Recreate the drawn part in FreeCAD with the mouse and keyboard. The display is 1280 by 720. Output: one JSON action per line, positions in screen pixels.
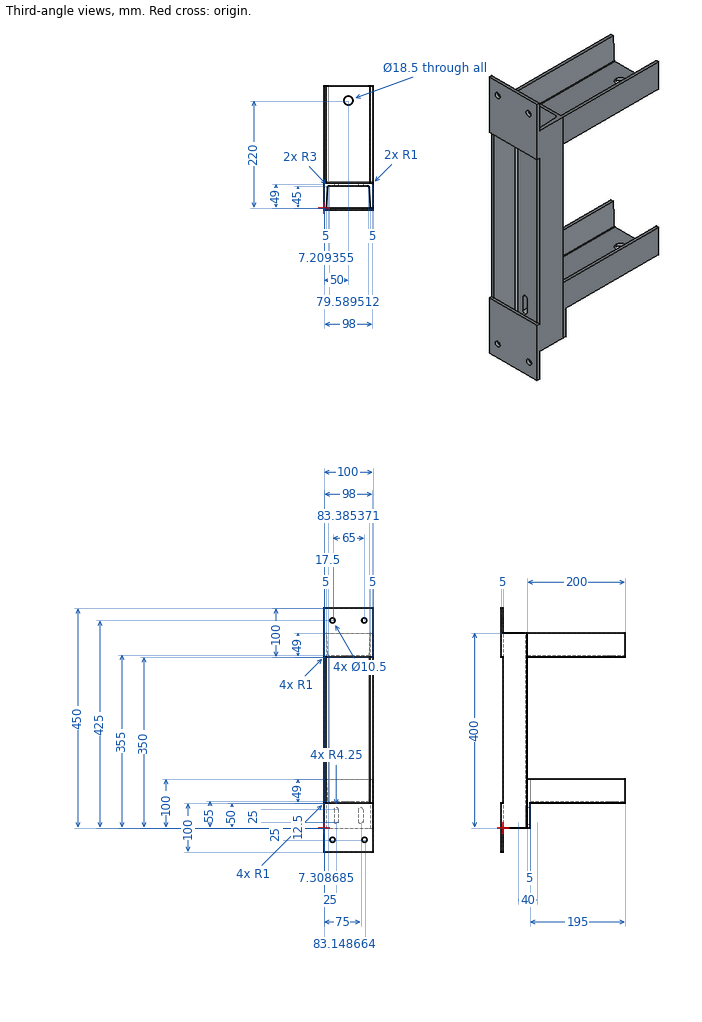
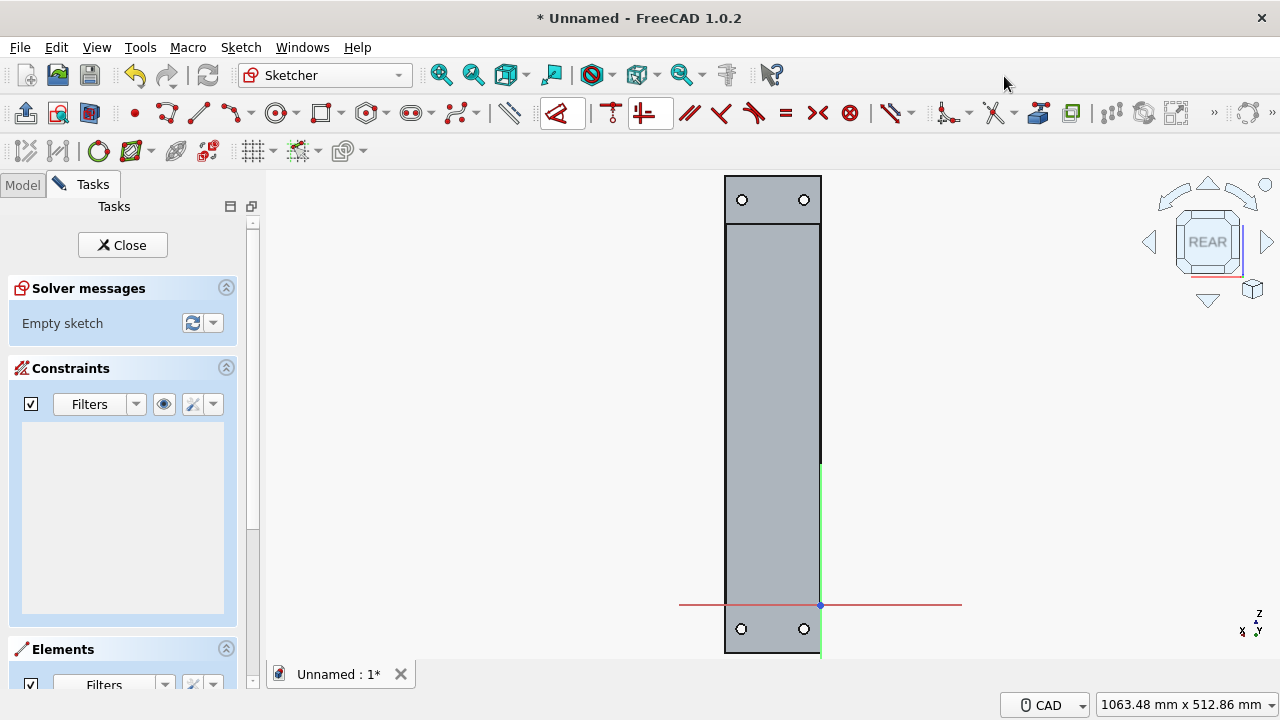
{"action": "scroll", "coordinate": [787, 215], "scroll_direction": "up", "scroll_amount": 9}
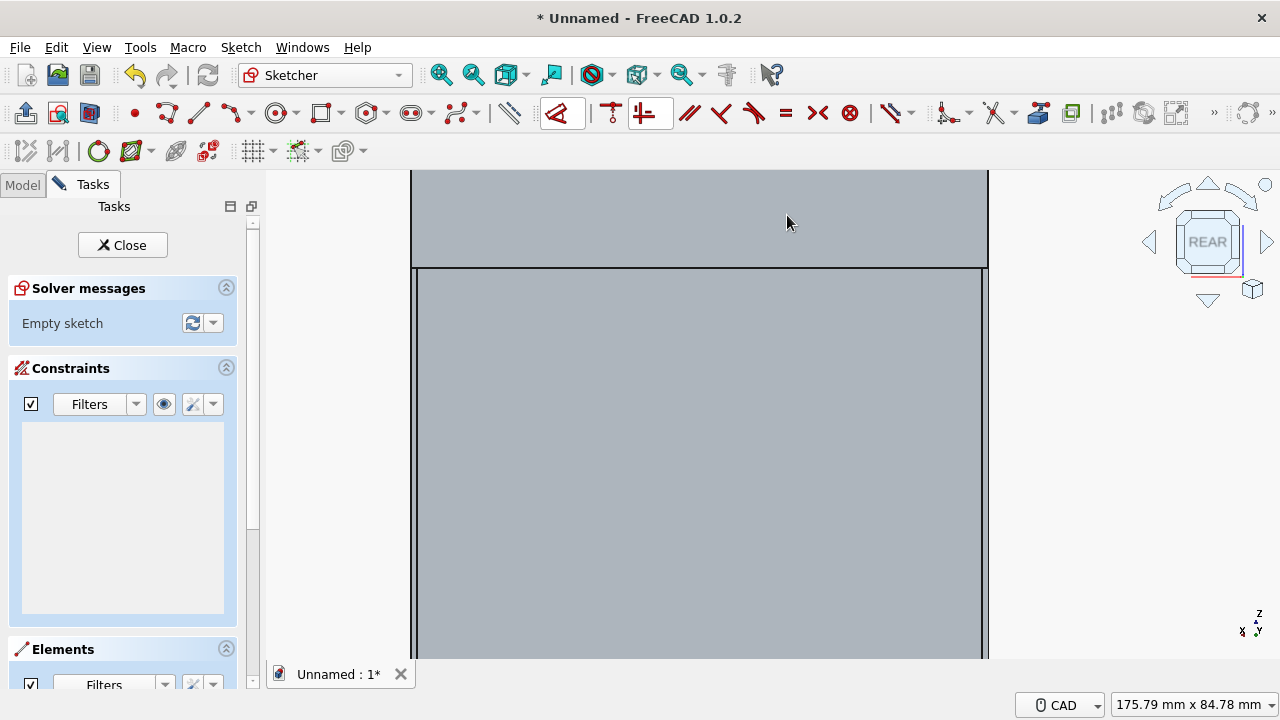
{"action": "key", "text": "g l"}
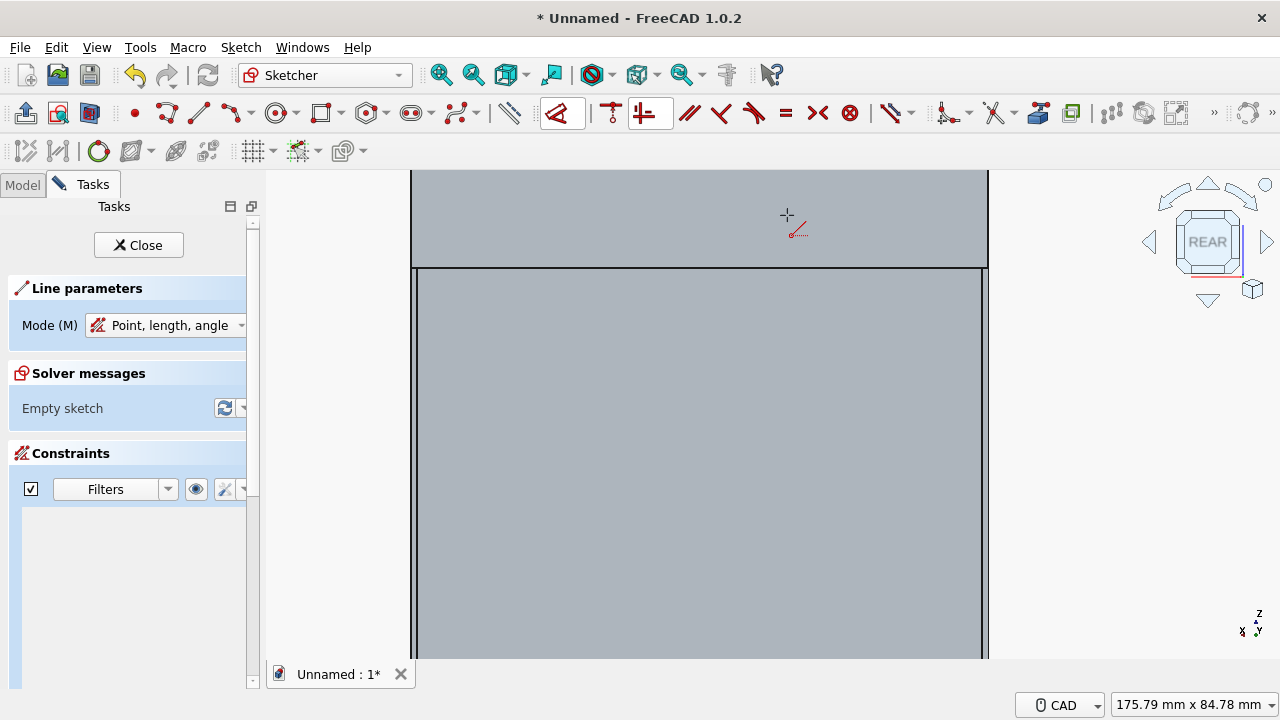
{"action": "left_click", "coordinate": [417, 556]}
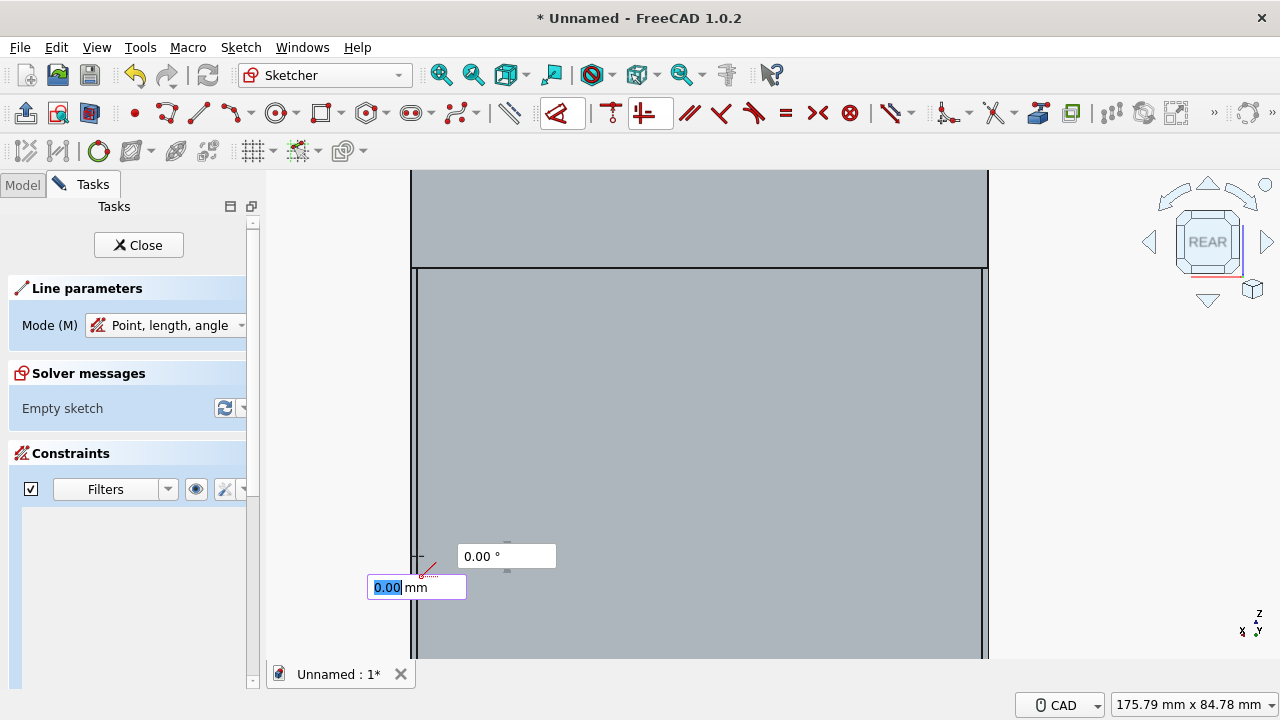
{"action": "scroll", "coordinate": [982, 556], "scroll_direction": "up", "scroll_amount": 6}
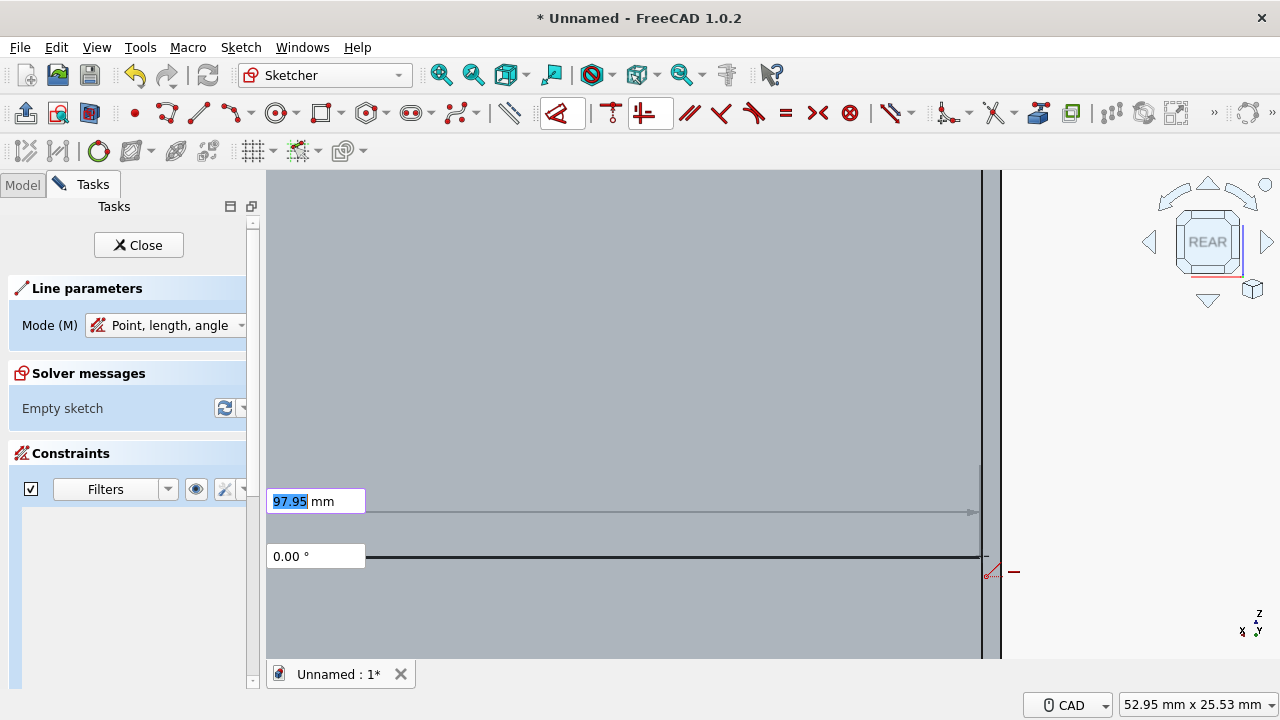
{"action": "left_click", "coordinate": [982, 554]}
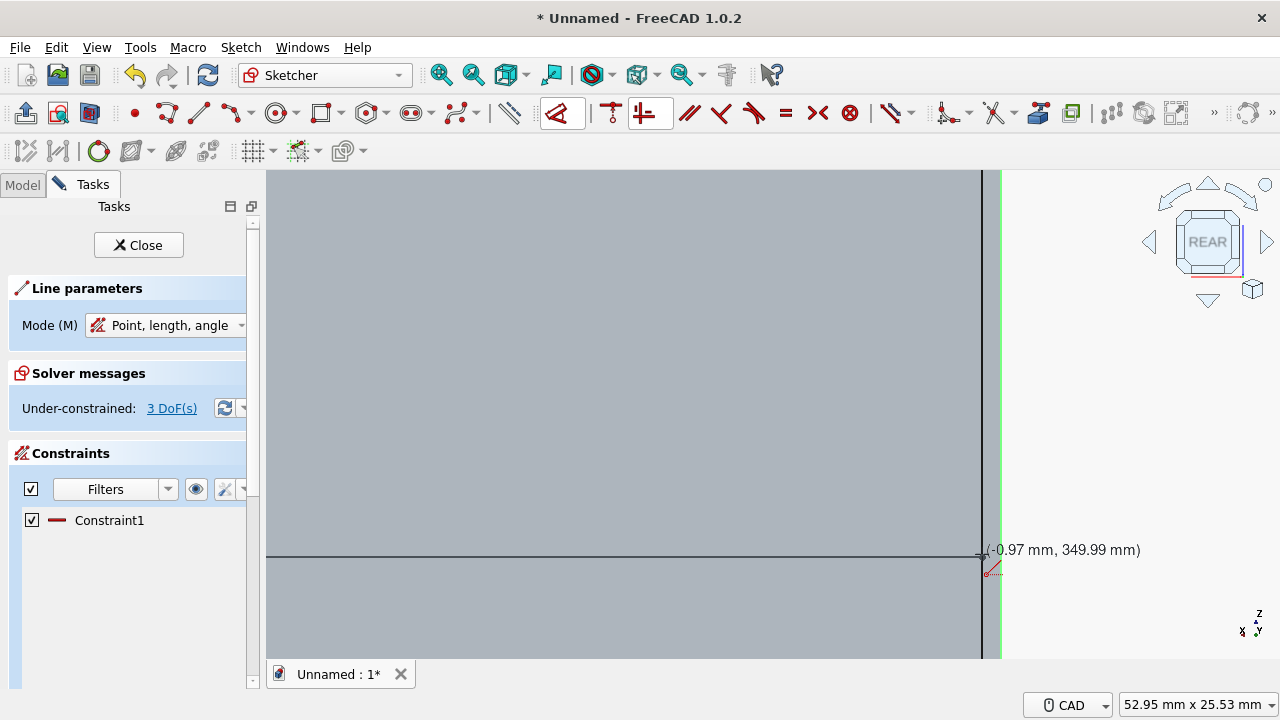
{"action": "key", "text": "g m"}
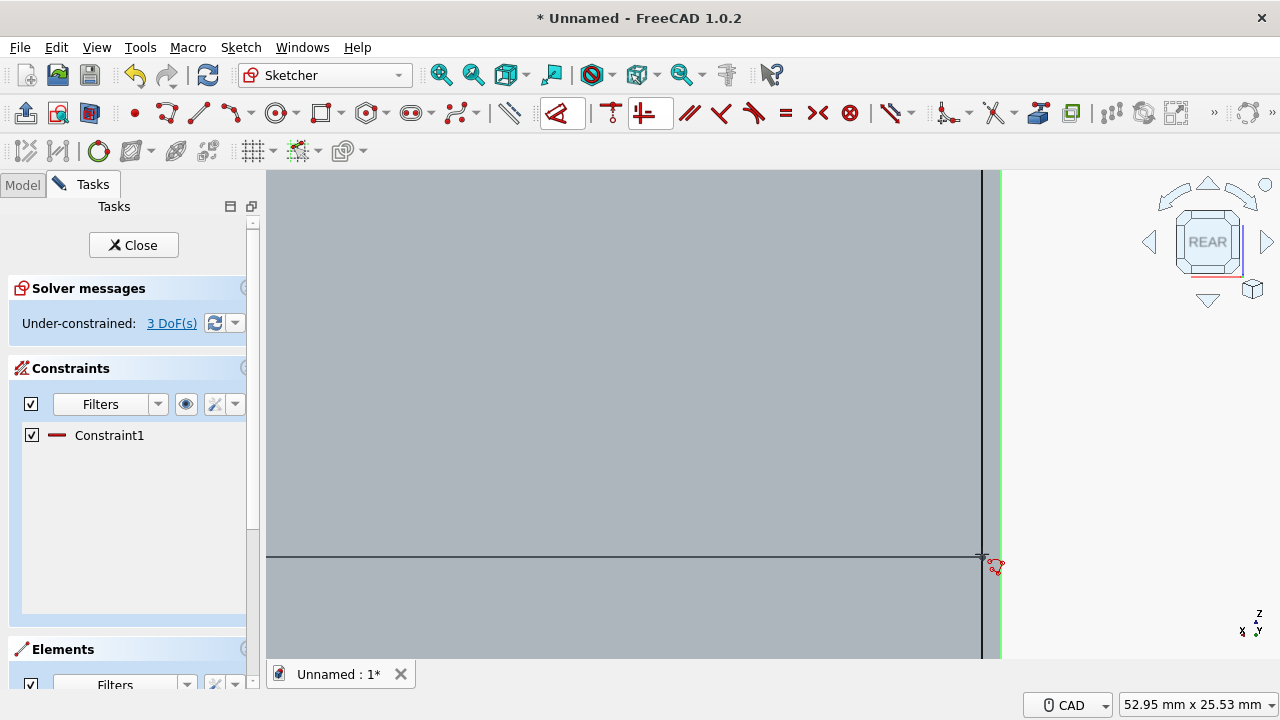
{"action": "left_click", "coordinate": [1001, 536]}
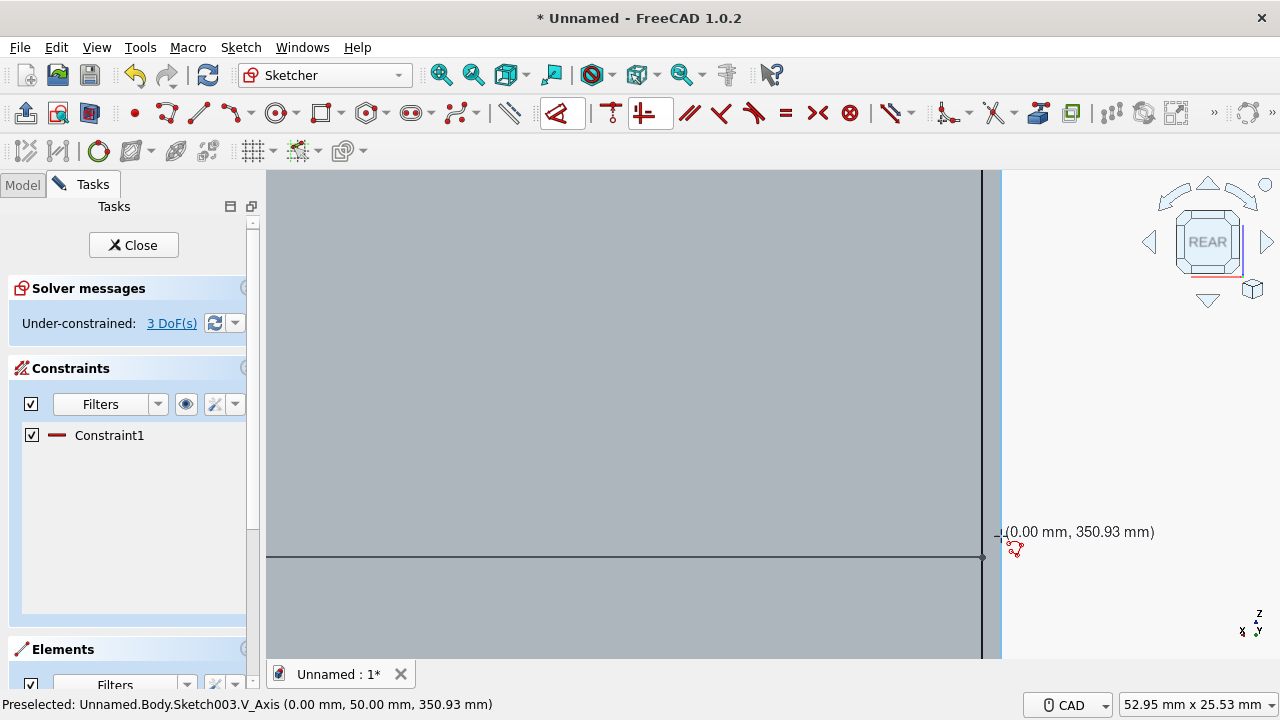
{"action": "scroll", "coordinate": [990, 560], "scroll_direction": "down", "scroll_amount": 6}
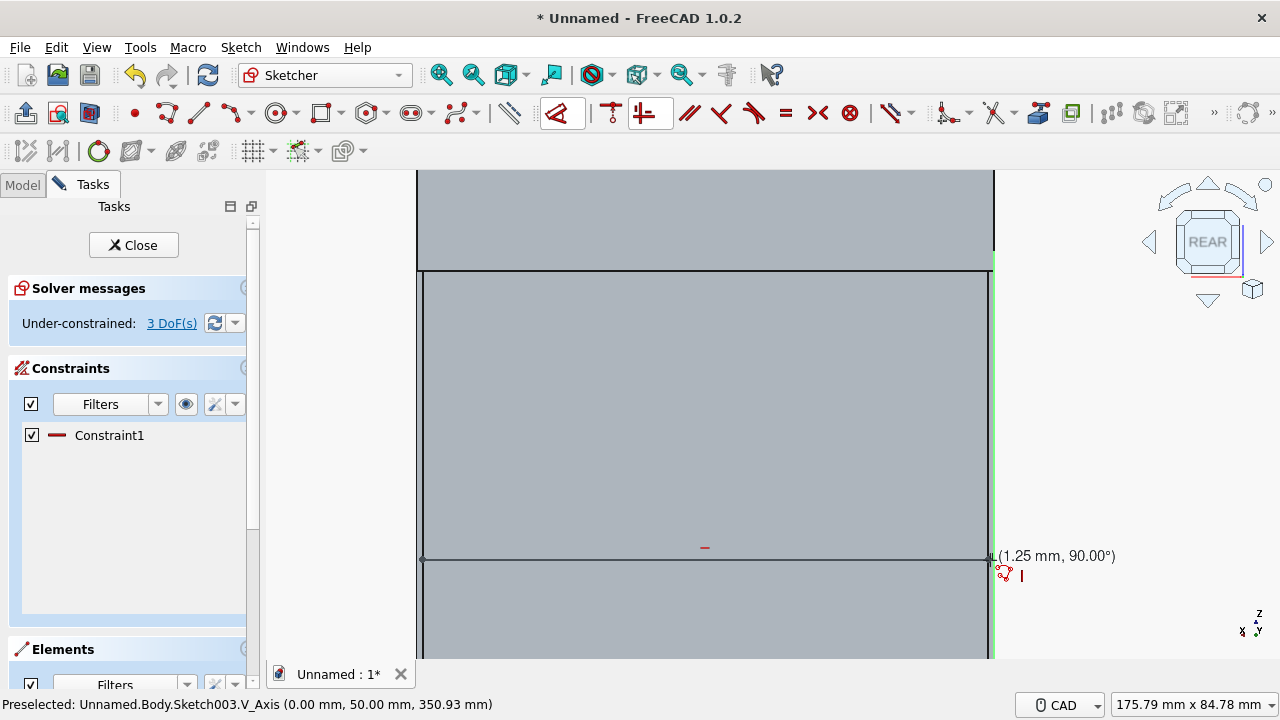
{"action": "left_click", "coordinate": [985, 271]}
{"action": "left_click", "coordinate": [965, 271]}
{"action": "left_click", "coordinate": [952, 525]}
{"action": "right_click", "coordinate": [952, 525]}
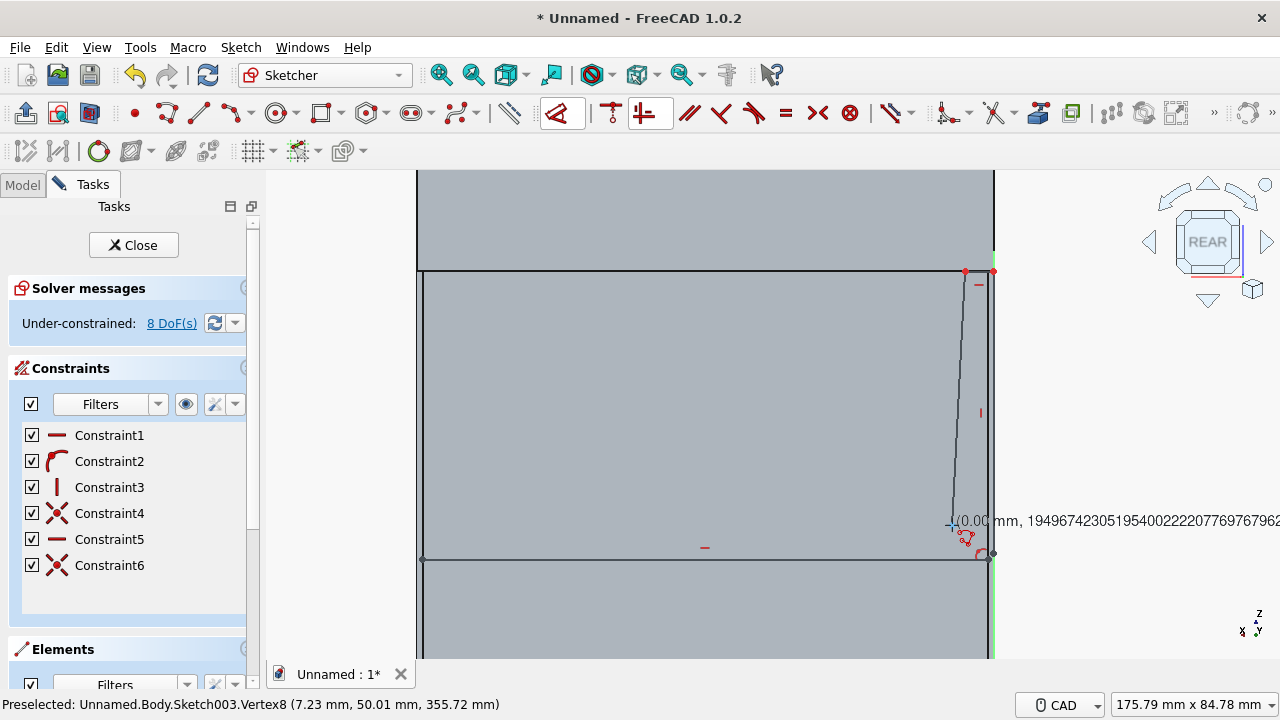
{"action": "left_click", "coordinate": [200, 114]}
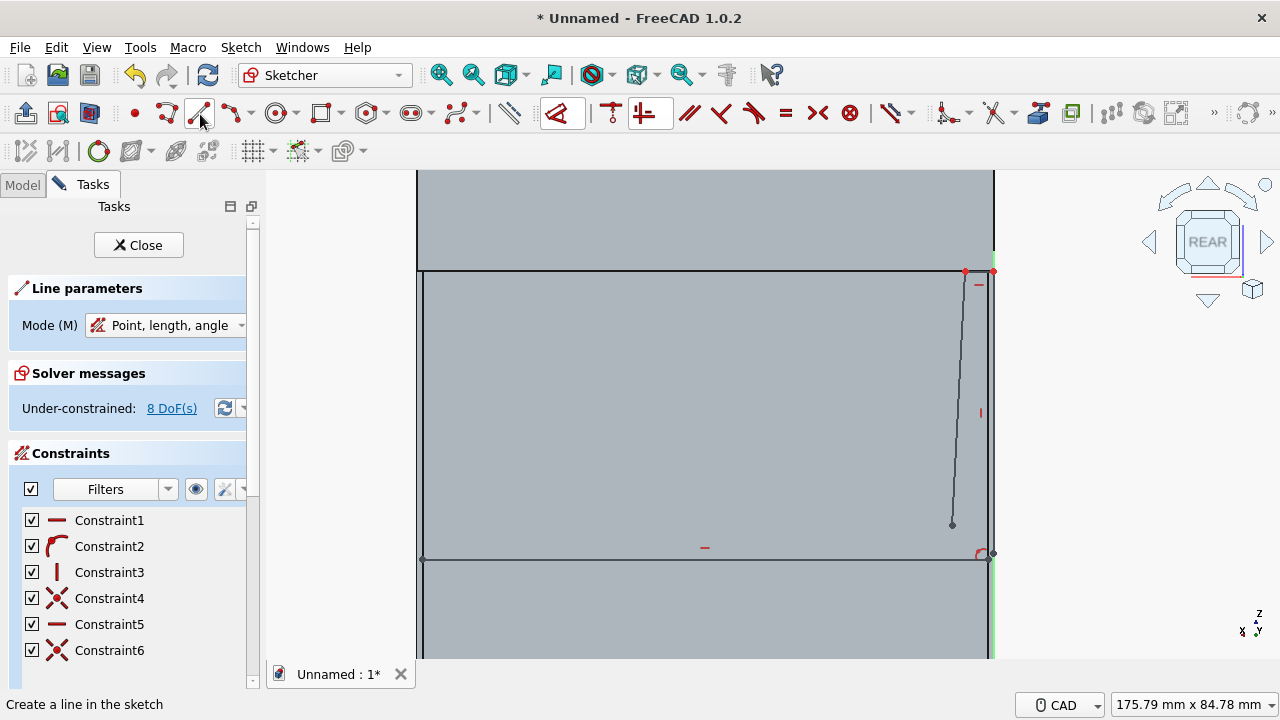
{"action": "scroll", "coordinate": [946, 530], "scroll_direction": "up", "scroll_amount": 4}